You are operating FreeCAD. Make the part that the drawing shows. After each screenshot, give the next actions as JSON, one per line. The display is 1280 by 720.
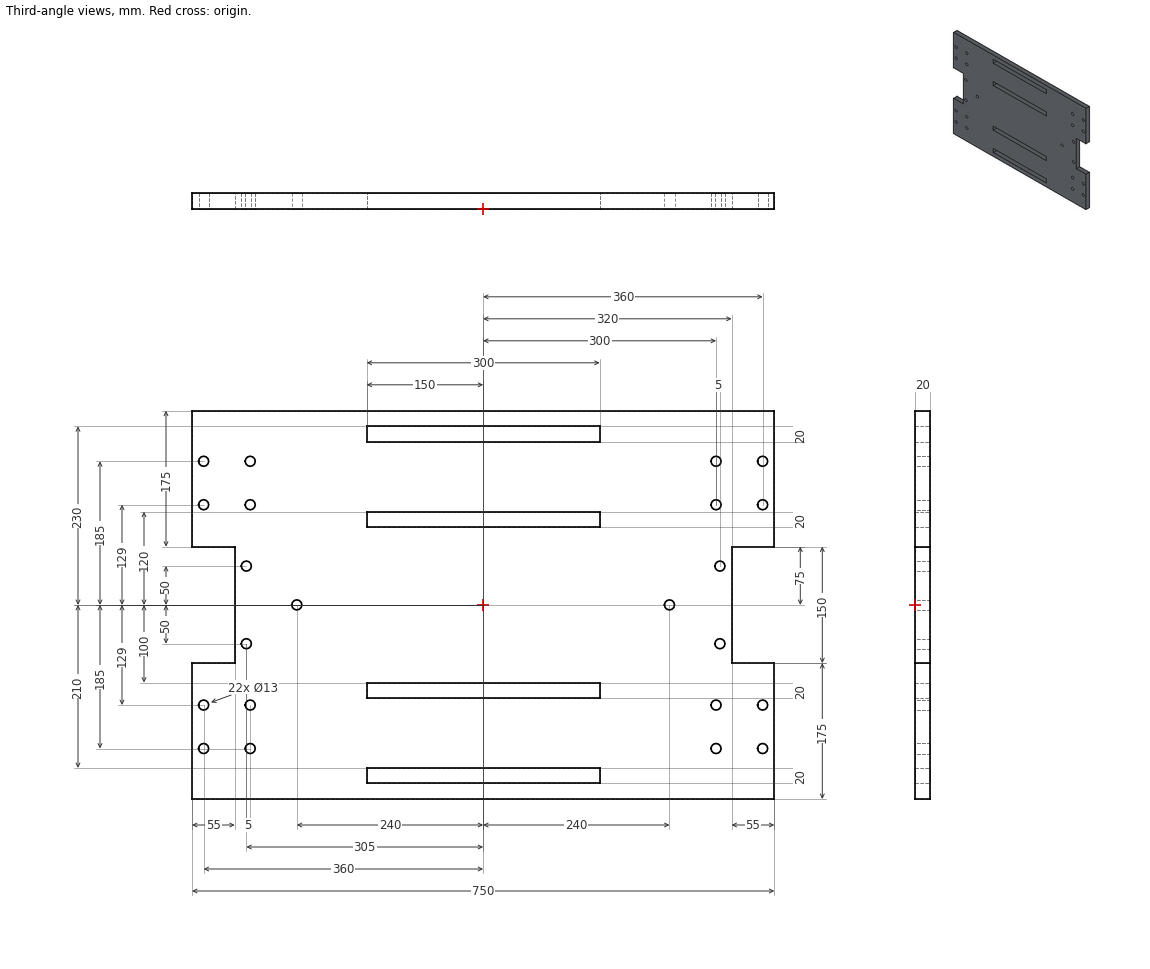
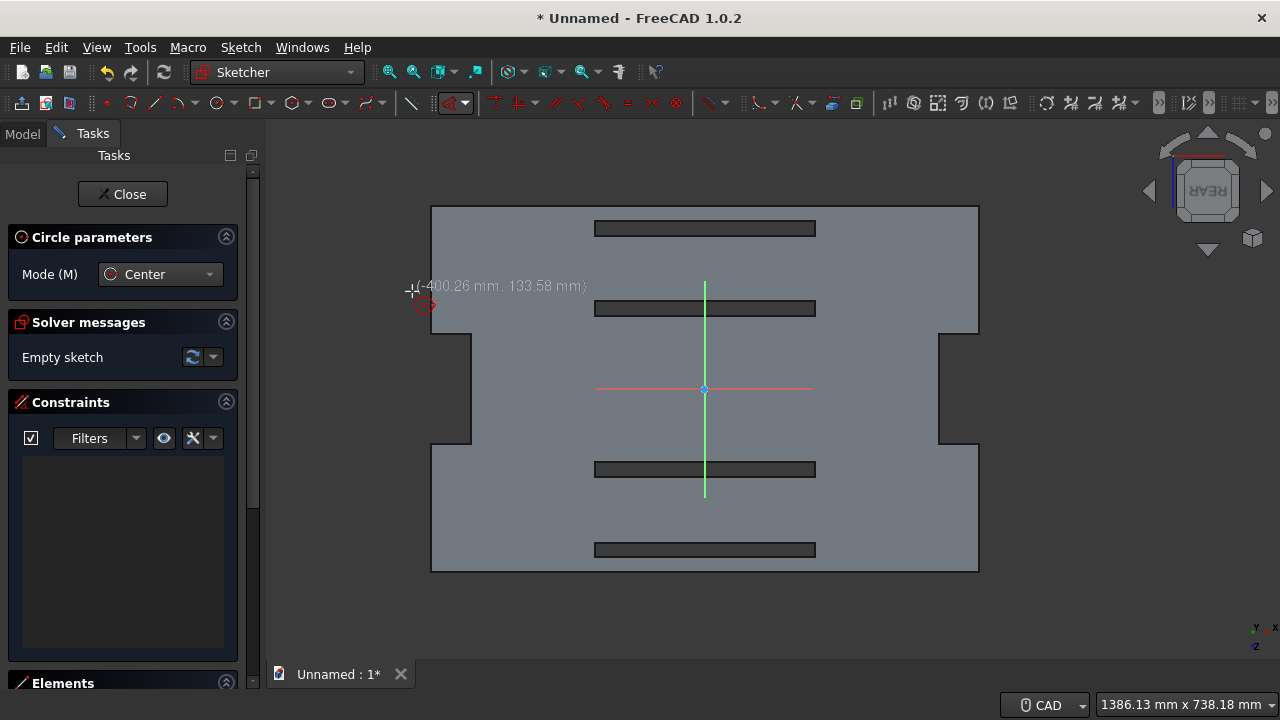
{"action": "left_click", "coordinate": [442, 295]}
{"action": "mouse_move", "coordinate": [445, 291]}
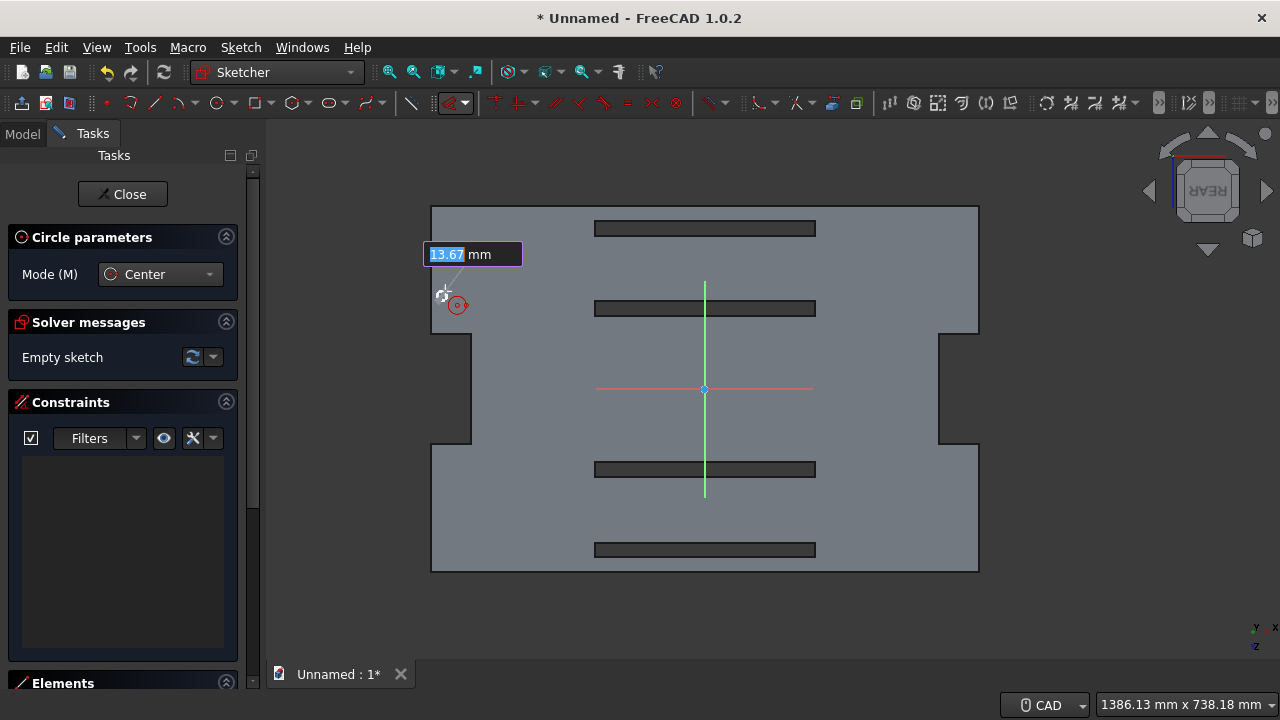
{"action": "type", "text": "13"}
{"action": "key", "text": "Return"}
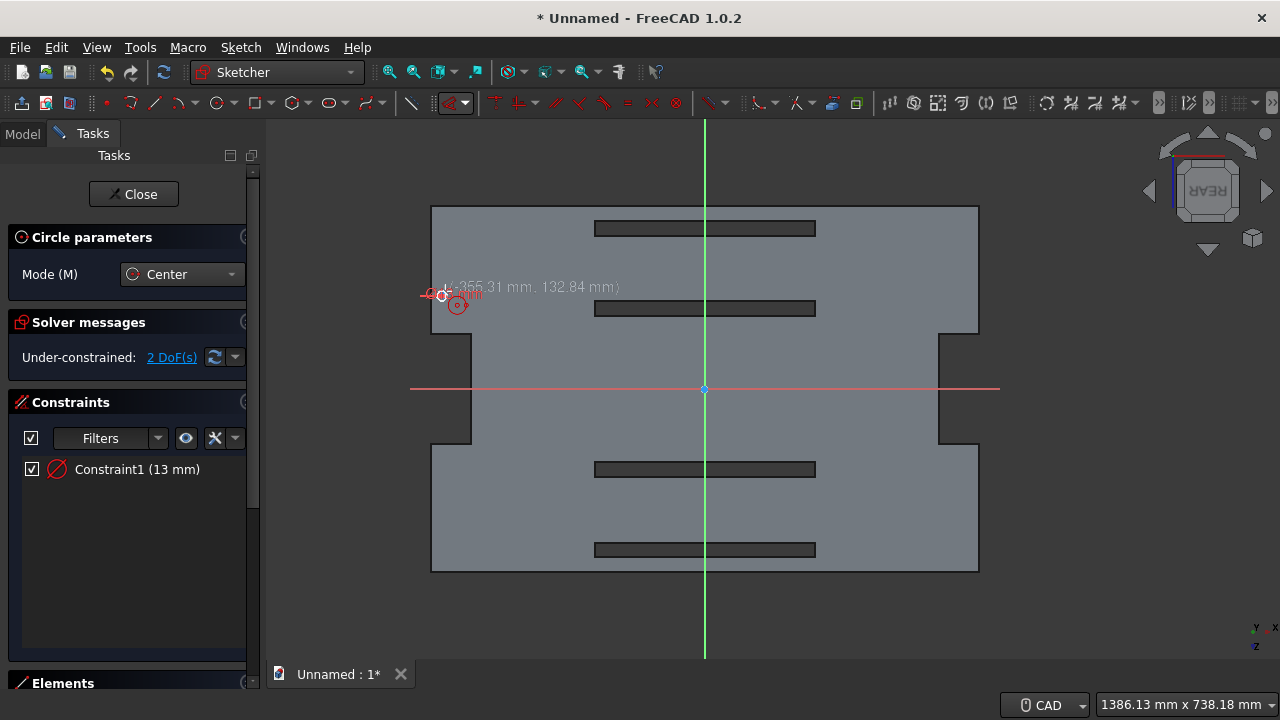
{"action": "scroll", "coordinate": [482, 353], "scroll_direction": "up", "scroll_amount": 8}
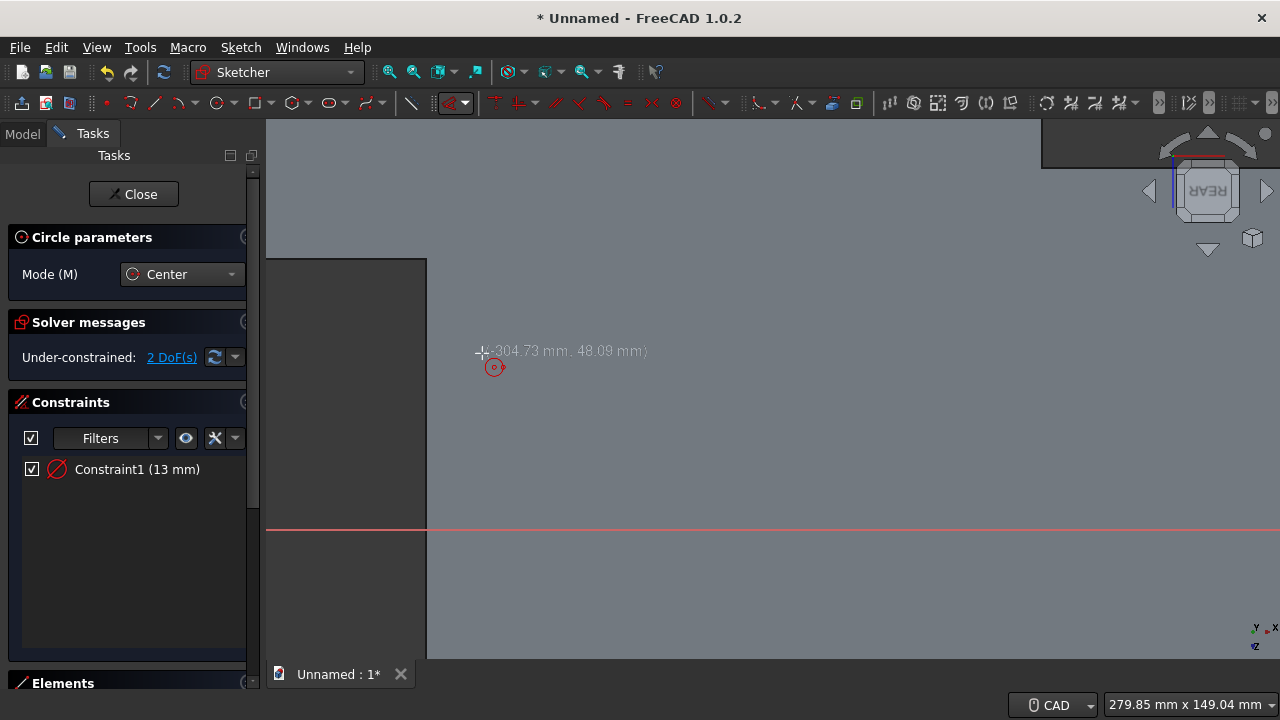
{"action": "scroll", "coordinate": [482, 353], "scroll_direction": "down", "scroll_amount": 8}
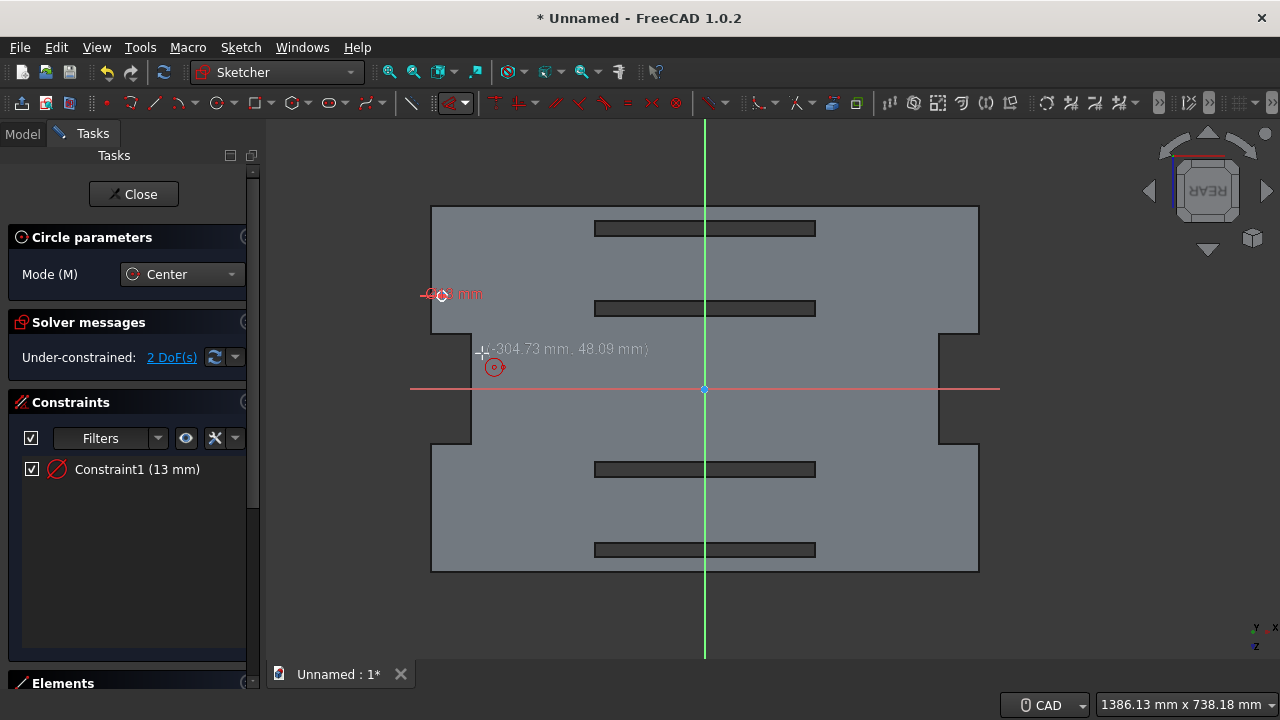
{"action": "left_click", "coordinate": [482, 353]}
{"action": "mouse_move", "coordinate": [485, 349]}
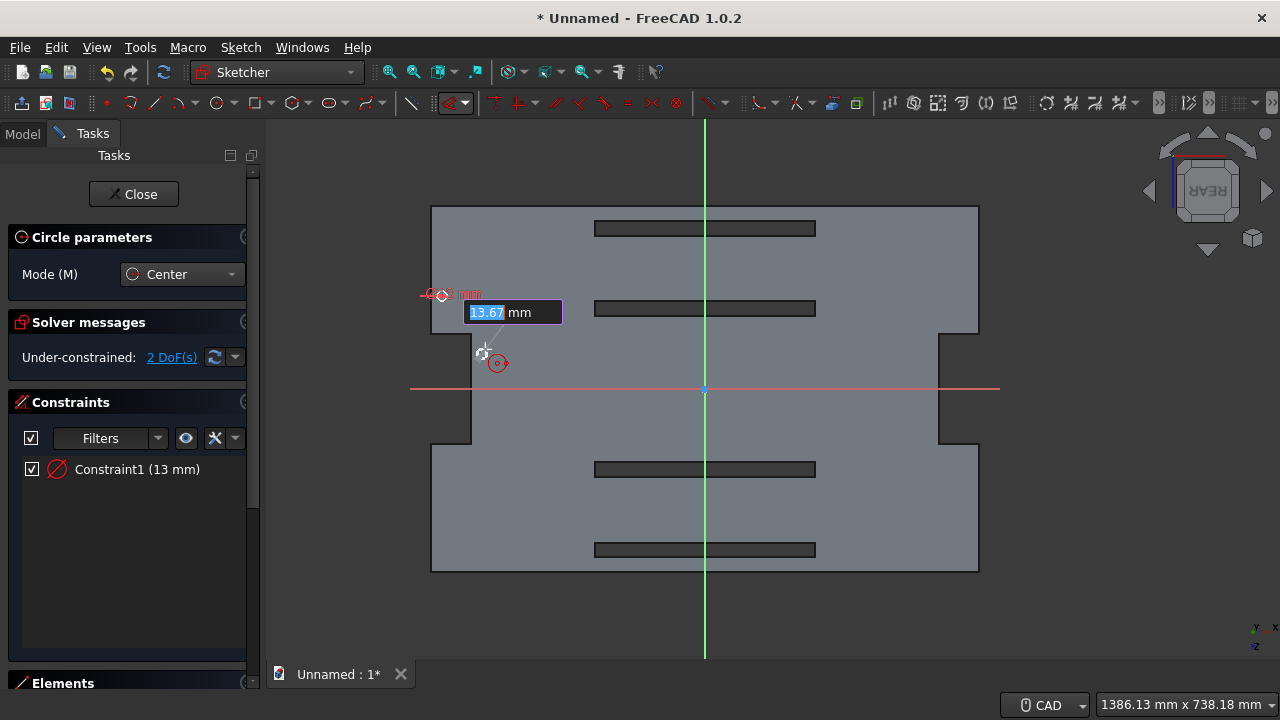
{"action": "type", "text": "13"}
{"action": "key", "text": "Return"}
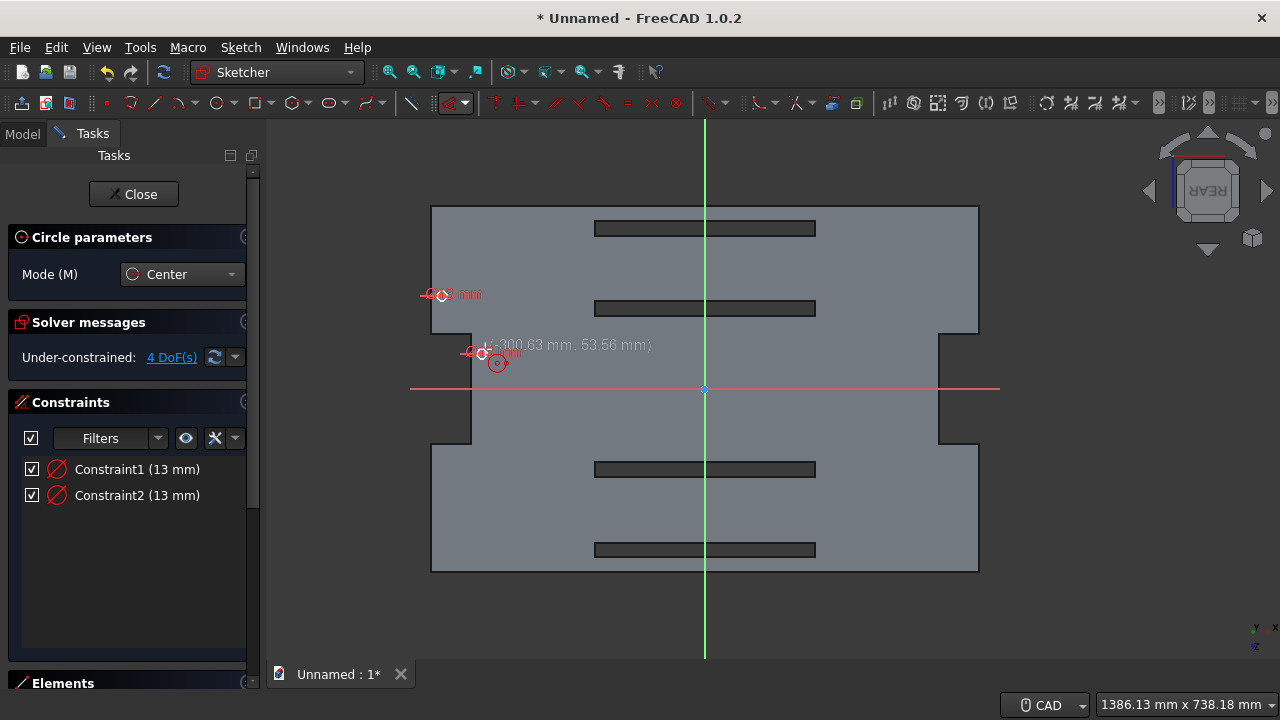
{"action": "scroll", "coordinate": [529, 389], "scroll_direction": "up", "scroll_amount": 8}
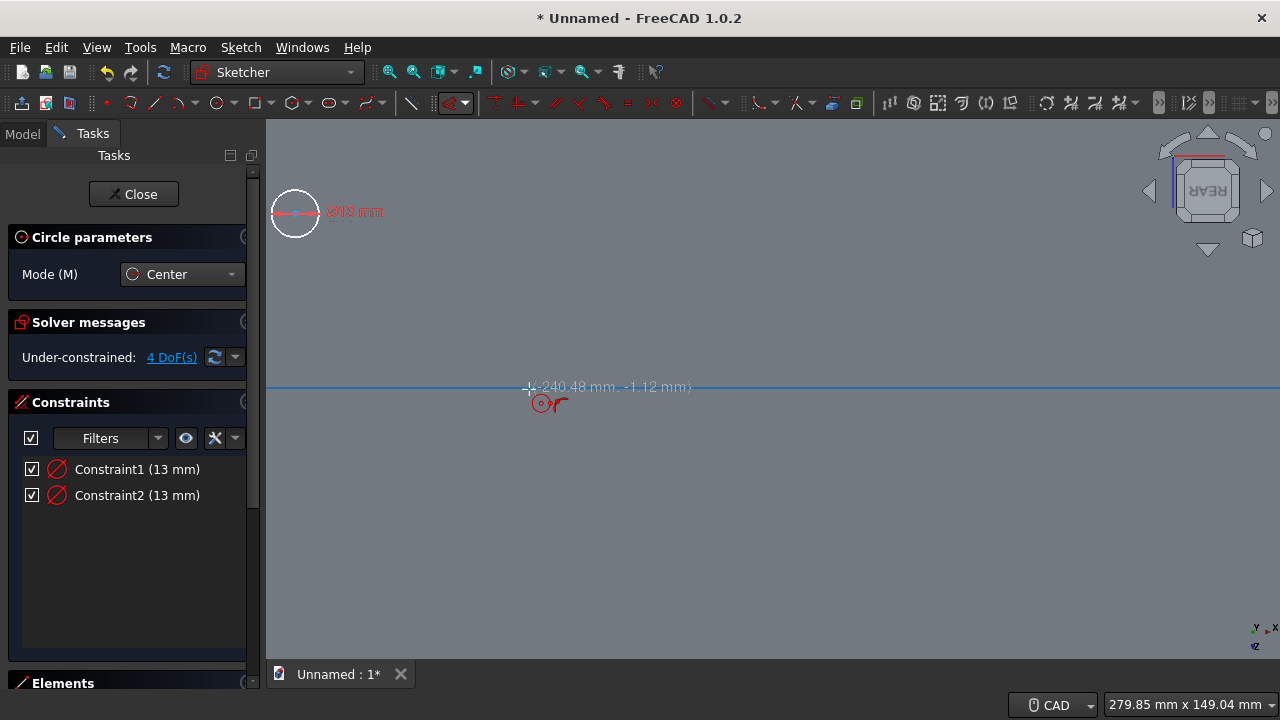
{"action": "scroll", "coordinate": [529, 389], "scroll_direction": "down", "scroll_amount": 8}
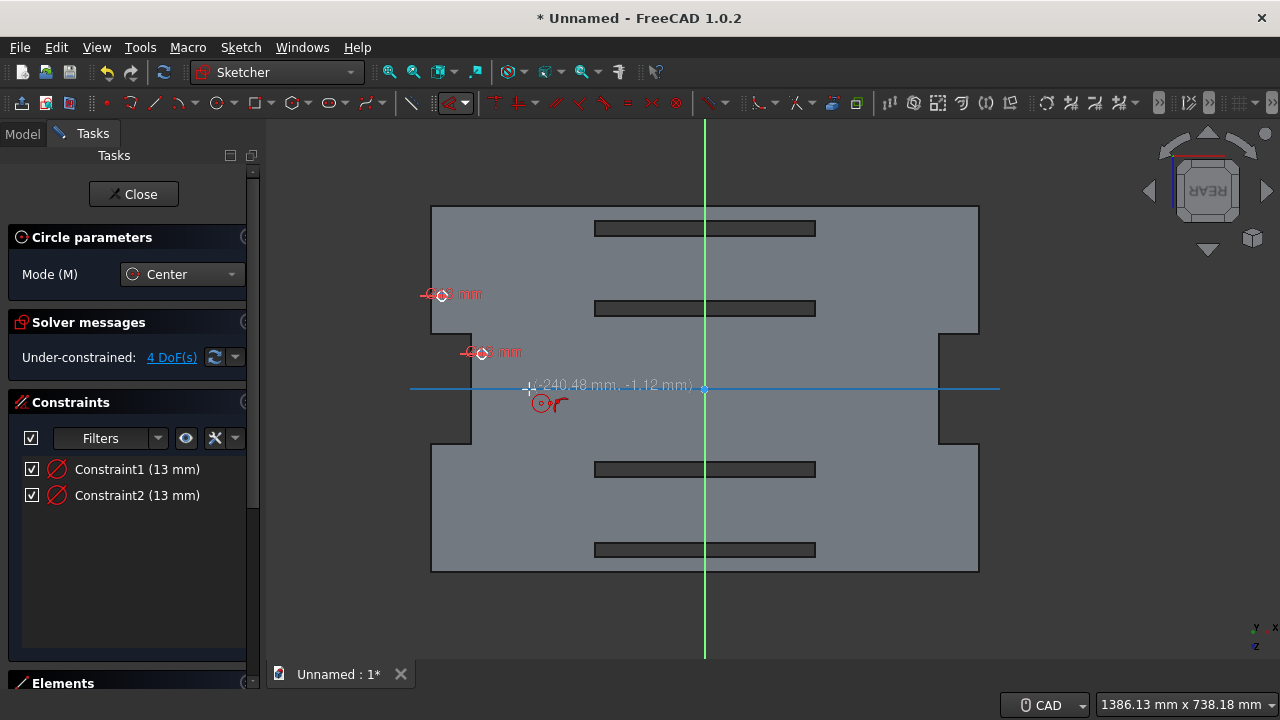
{"action": "left_click", "coordinate": [529, 389]}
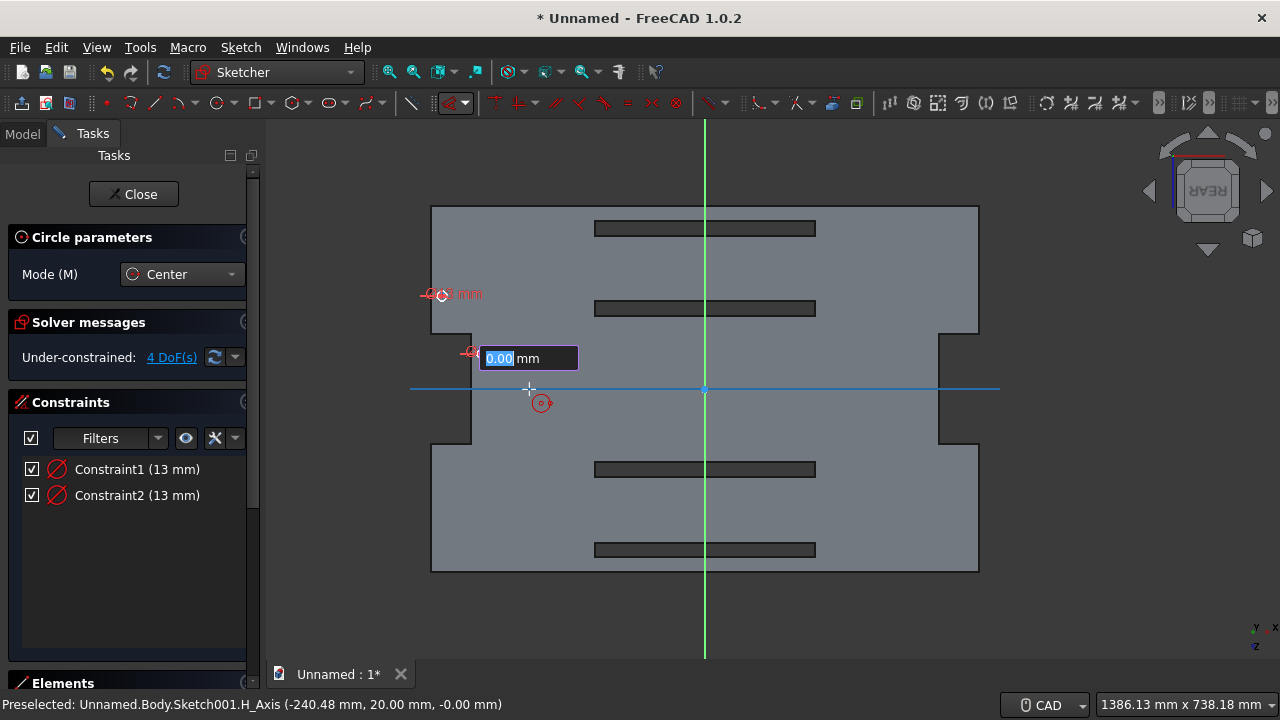
{"action": "scroll", "coordinate": [528, 394], "scroll_direction": "up", "scroll_amount": 7}
{"action": "mouse_move", "coordinate": [526, 391]}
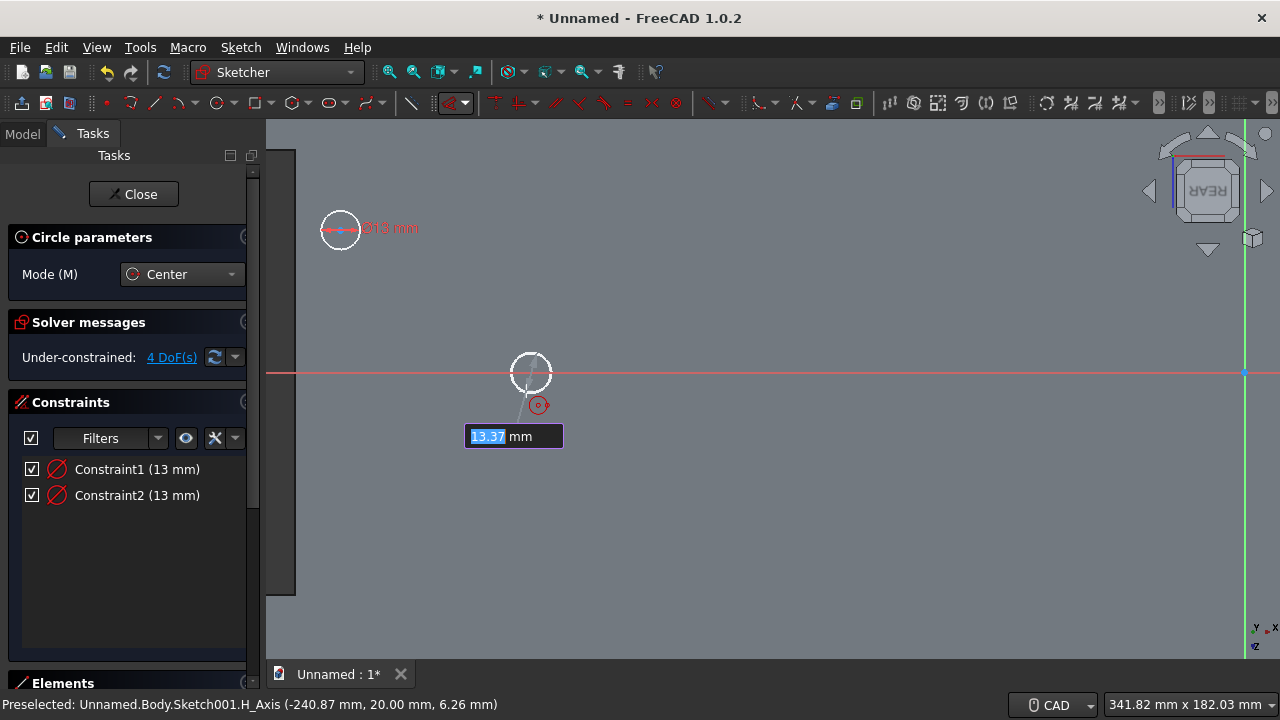
{"action": "type", "text": "13"}
{"action": "key", "text": "Return"}